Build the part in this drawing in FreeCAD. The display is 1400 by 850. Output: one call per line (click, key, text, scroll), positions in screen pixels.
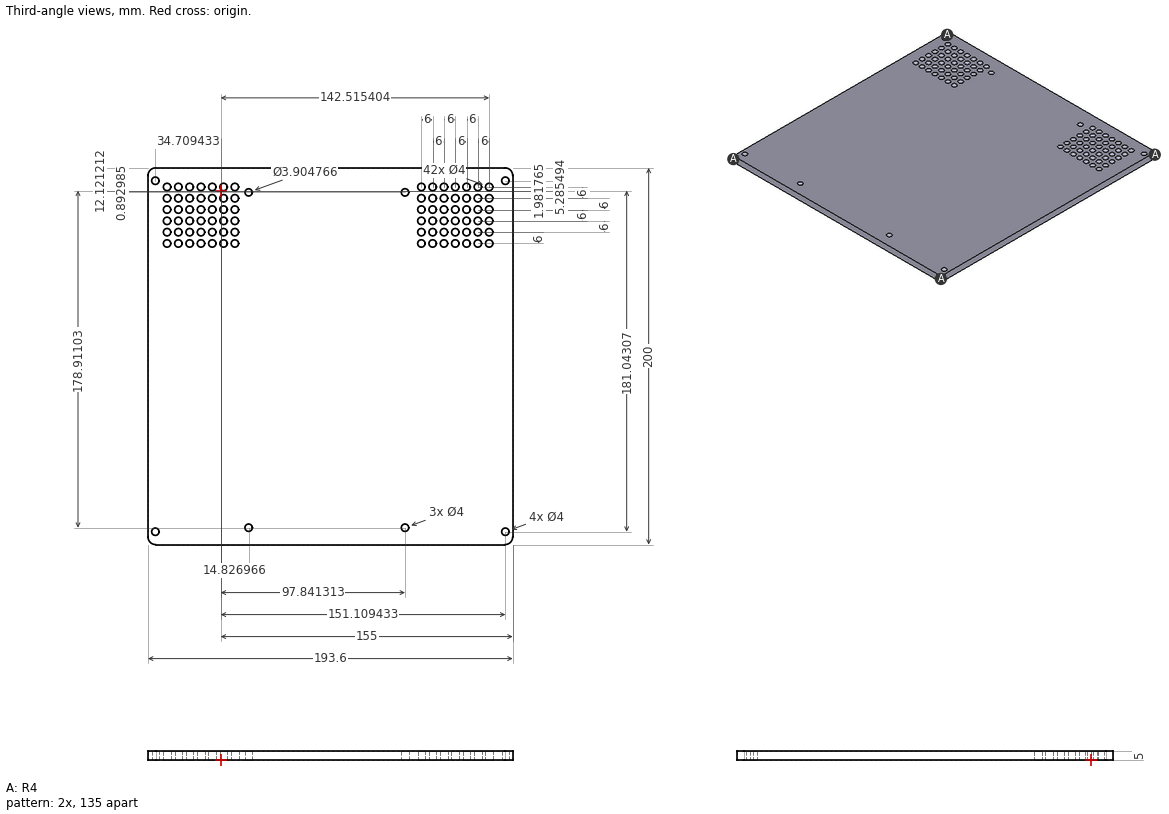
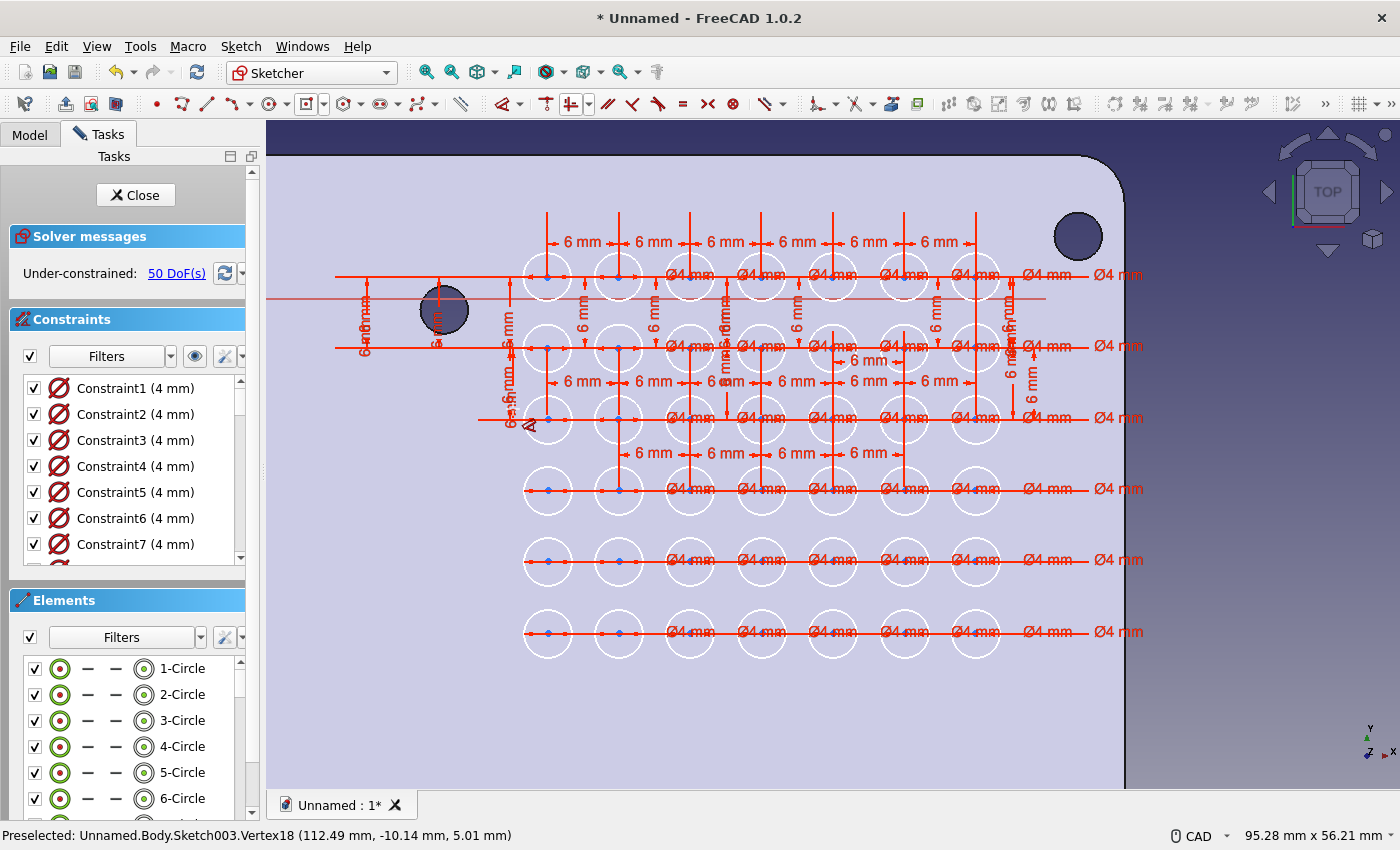
click(619, 420)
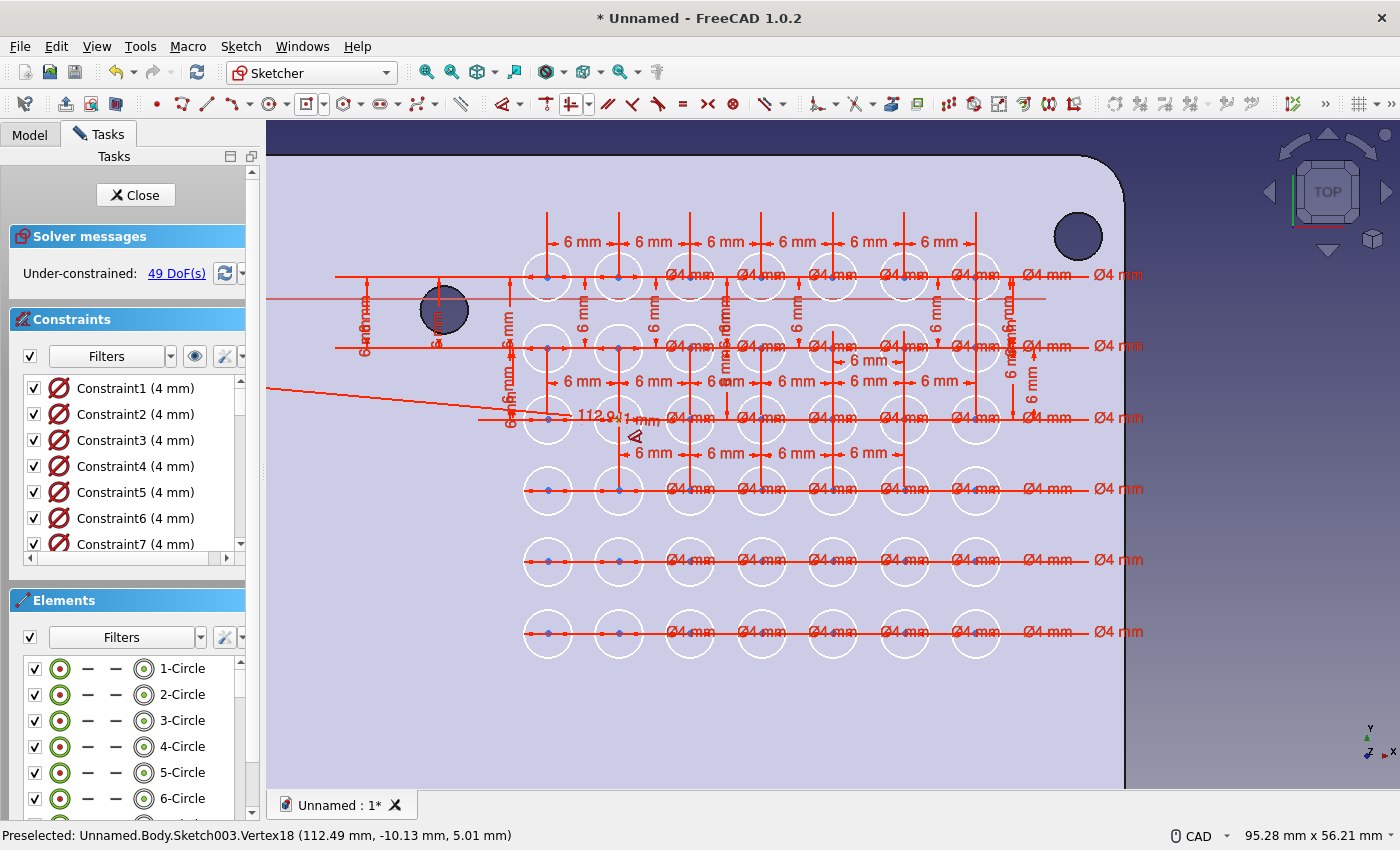
click(548, 420)
click(583, 454)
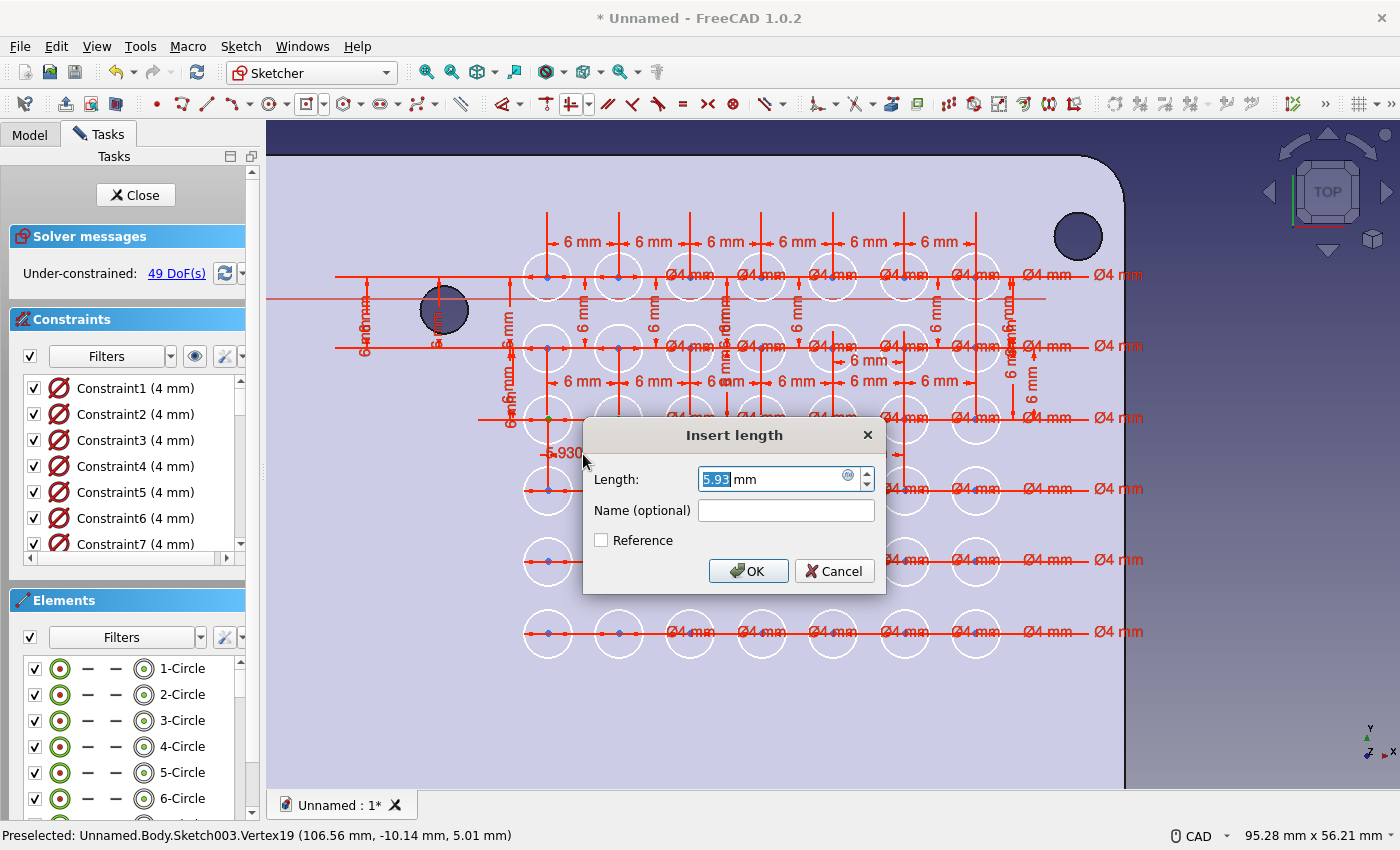
text(6)
key(Return)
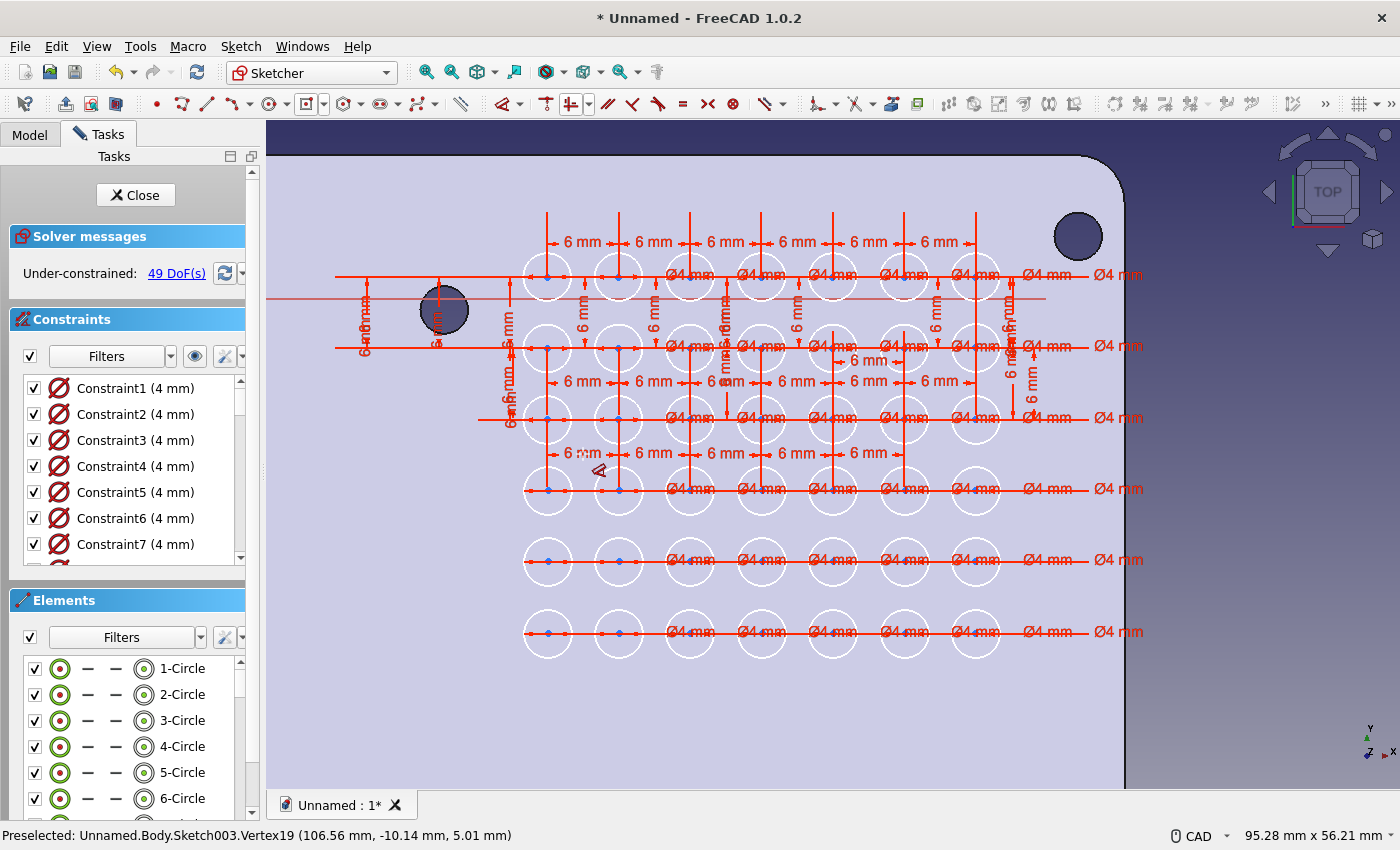
click(547, 348)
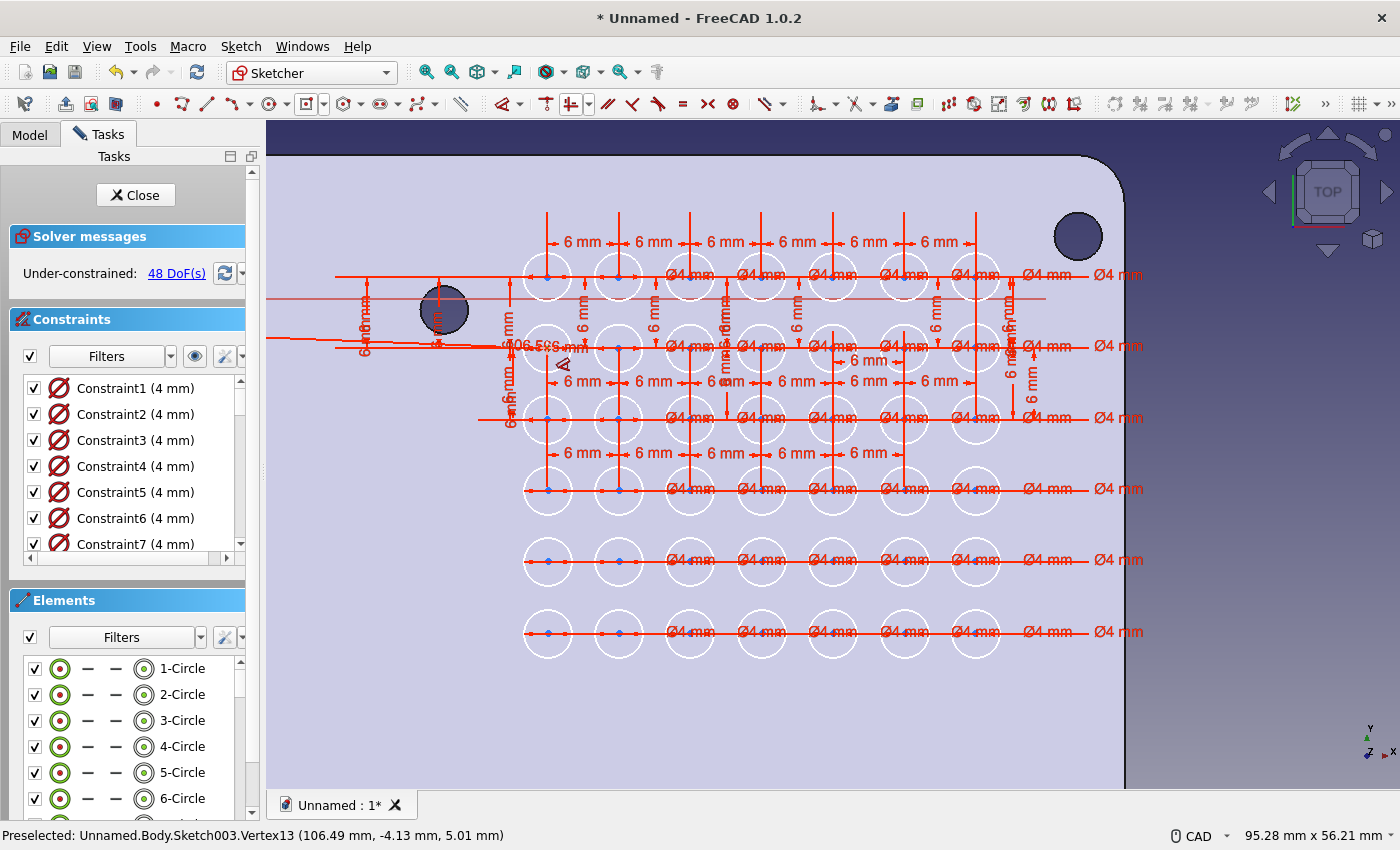
click(547, 420)
click(489, 359)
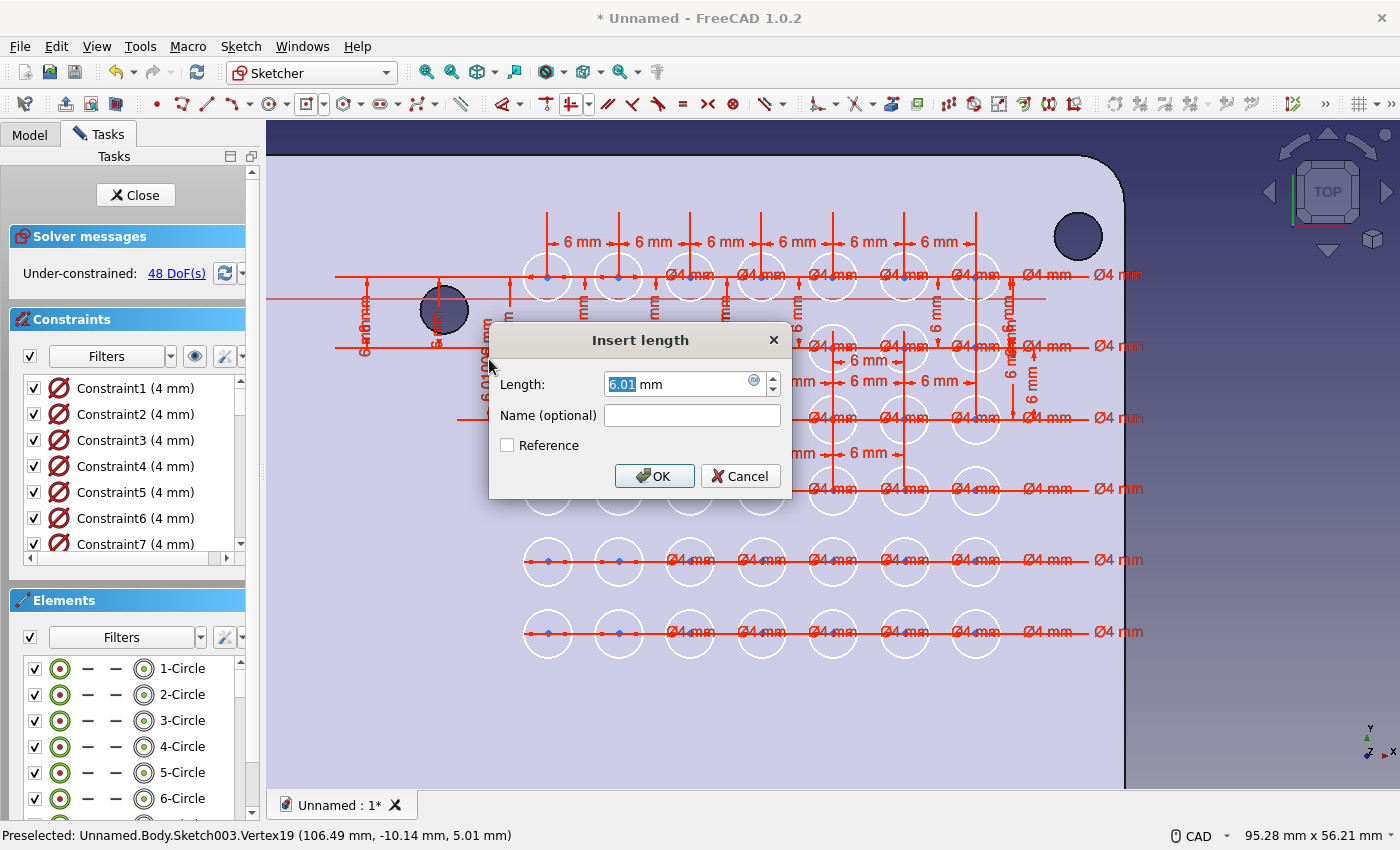
text(6)
key(Return)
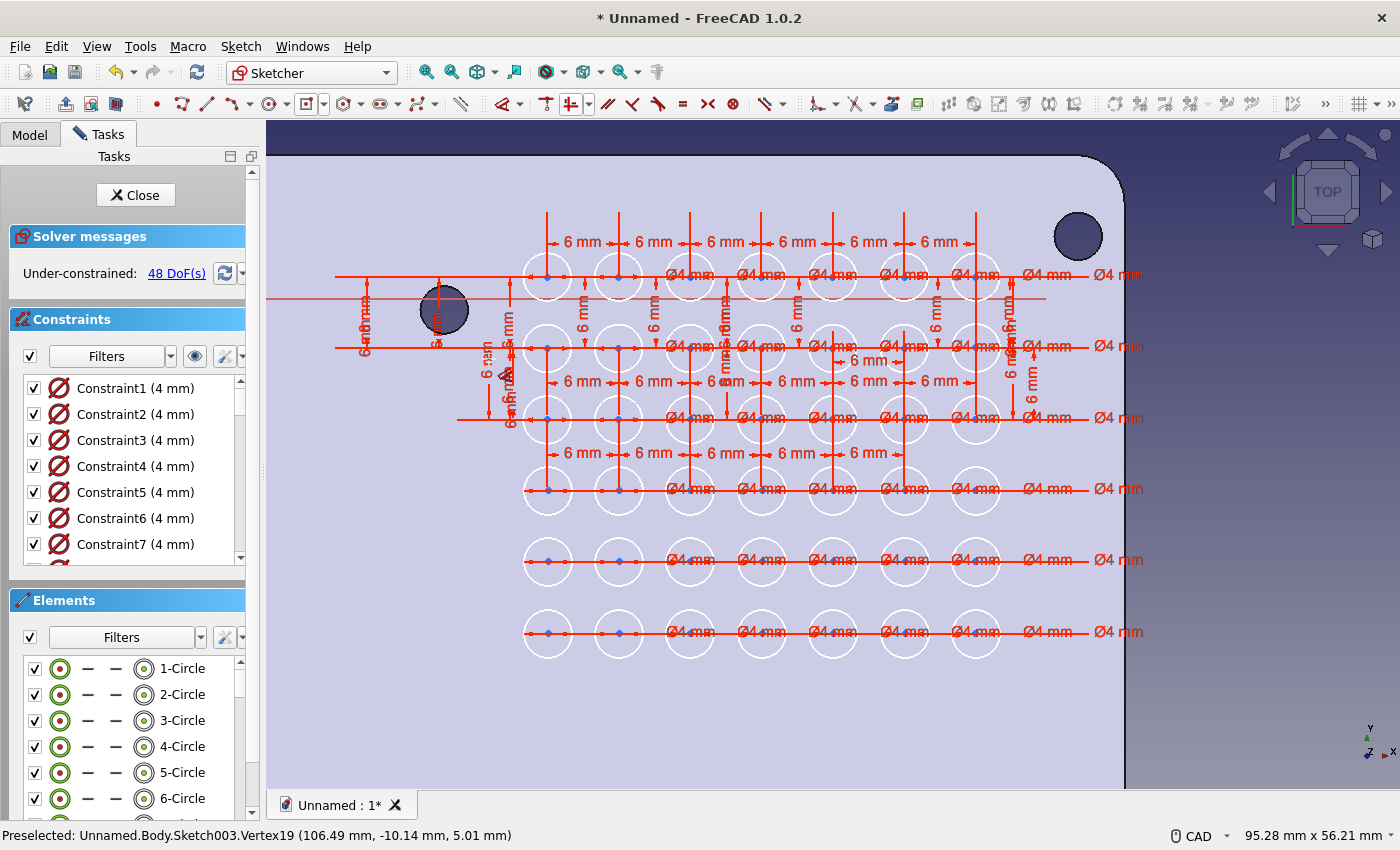
click(833, 420)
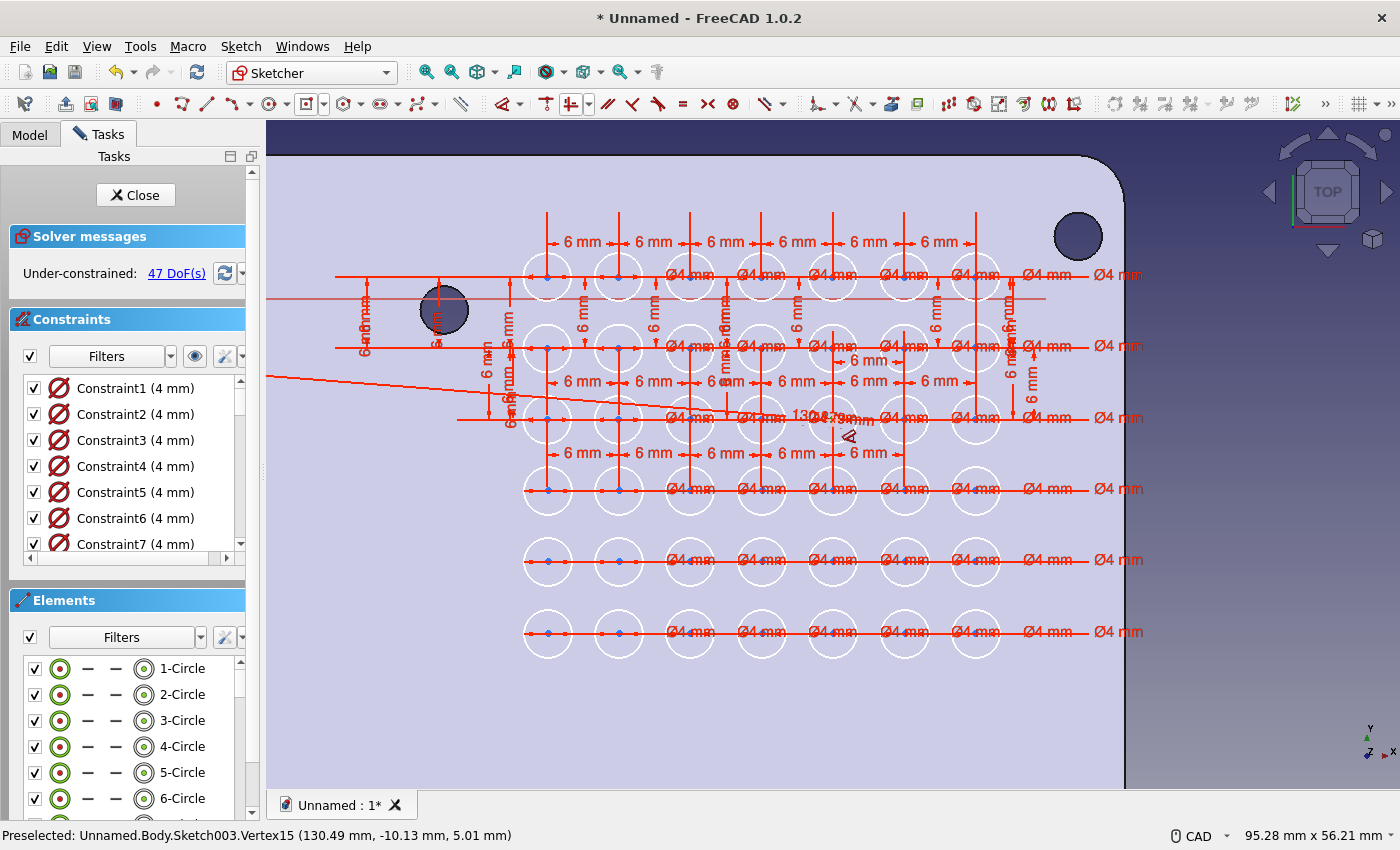
click(905, 491)
click(869, 525)